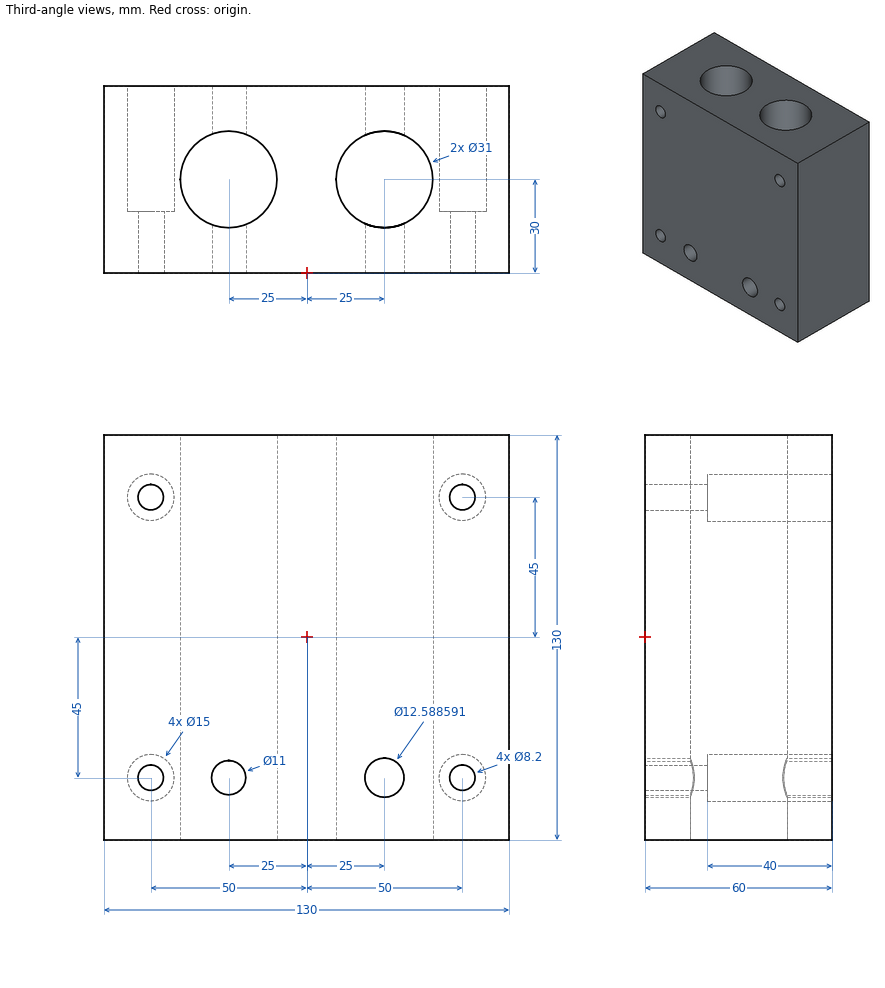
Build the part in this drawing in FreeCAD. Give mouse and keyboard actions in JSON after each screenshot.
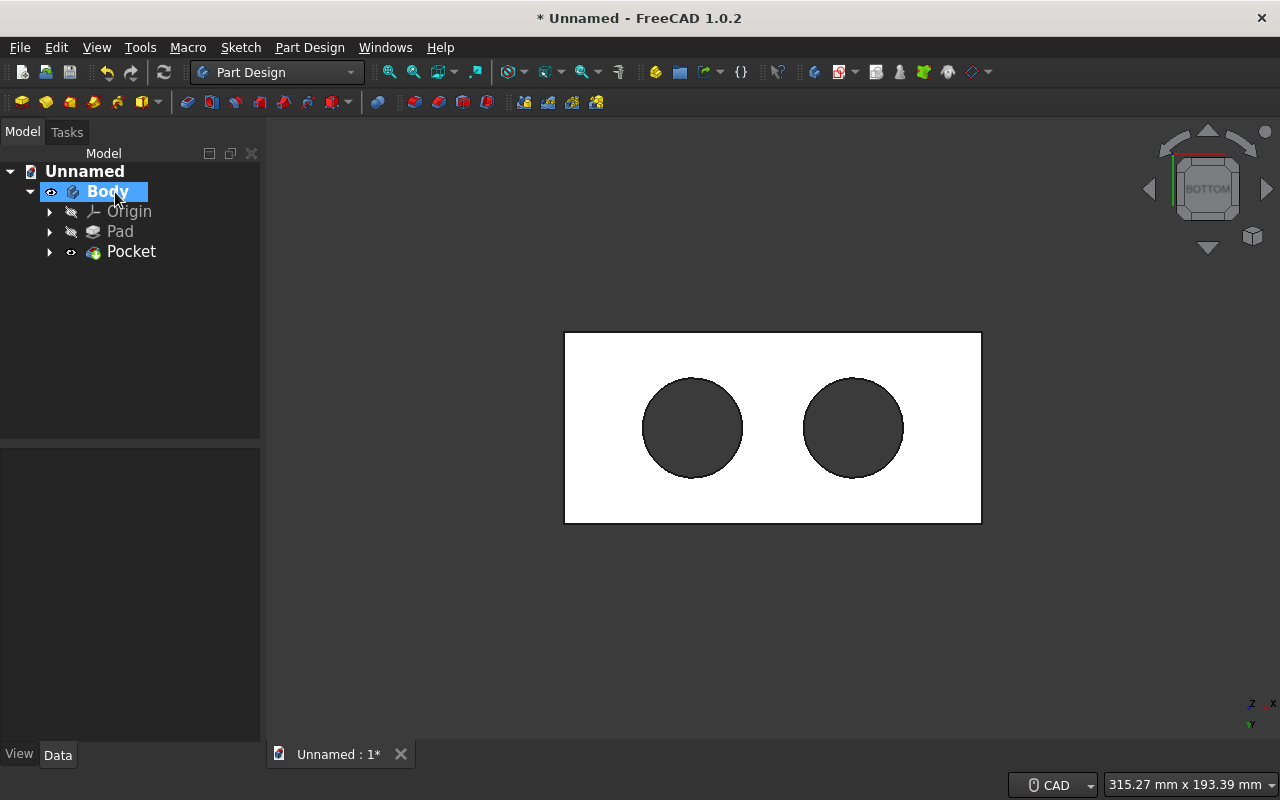
{"action": "key", "text": "4"}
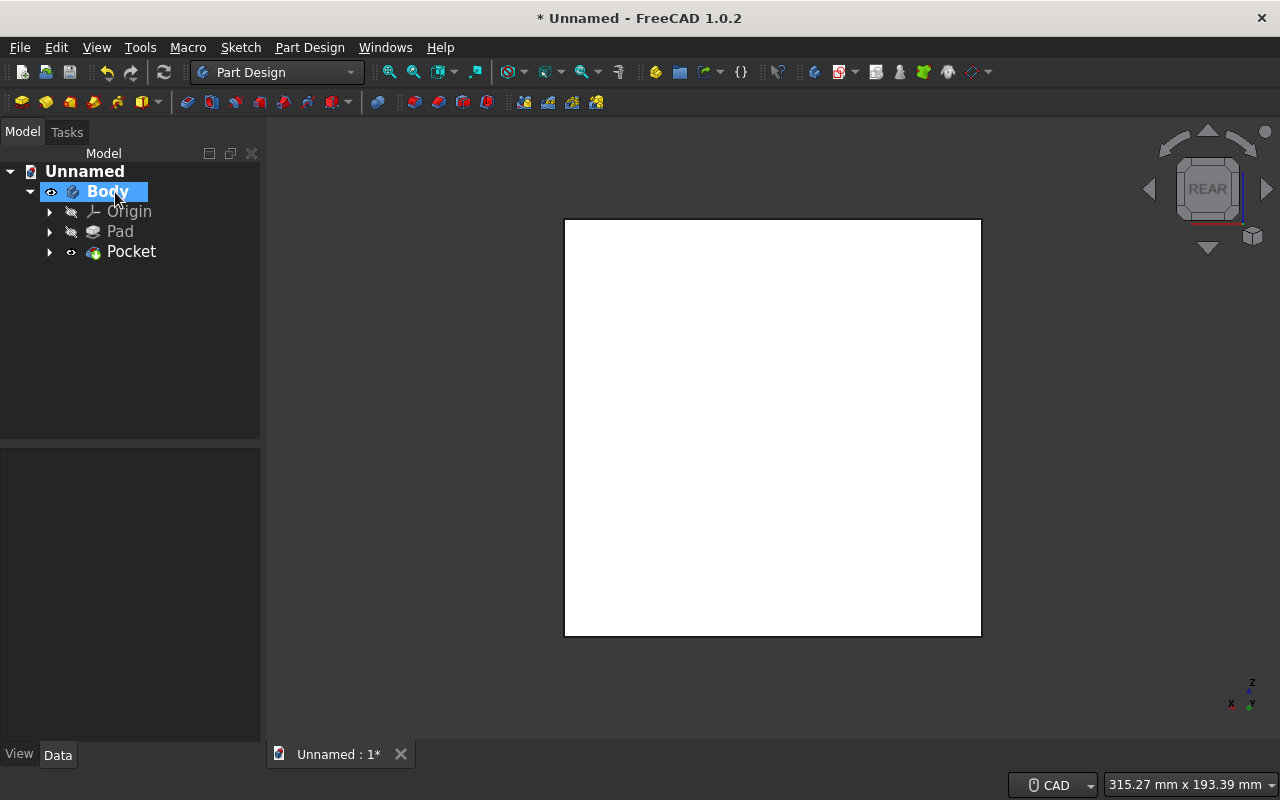
{"action": "left_click", "coordinate": [773, 427]}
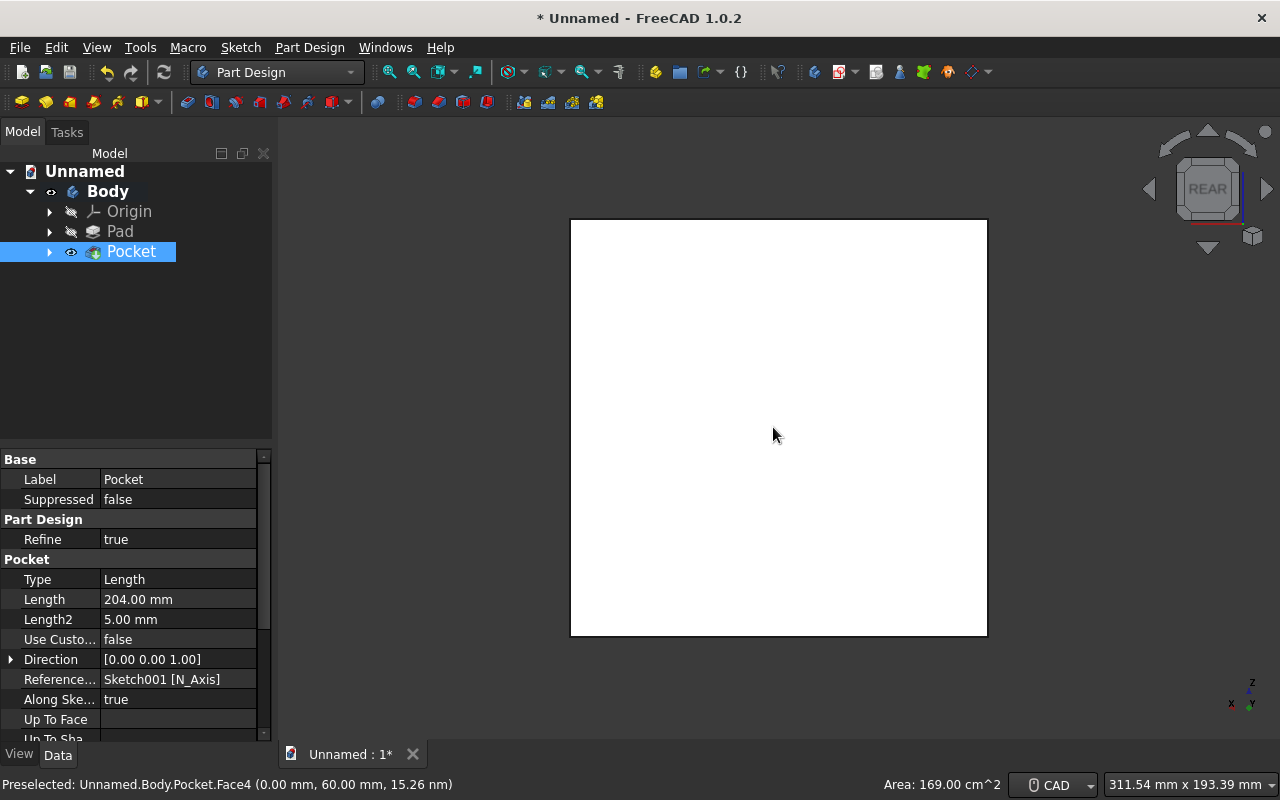
{"action": "left_click", "coordinate": [840, 72]}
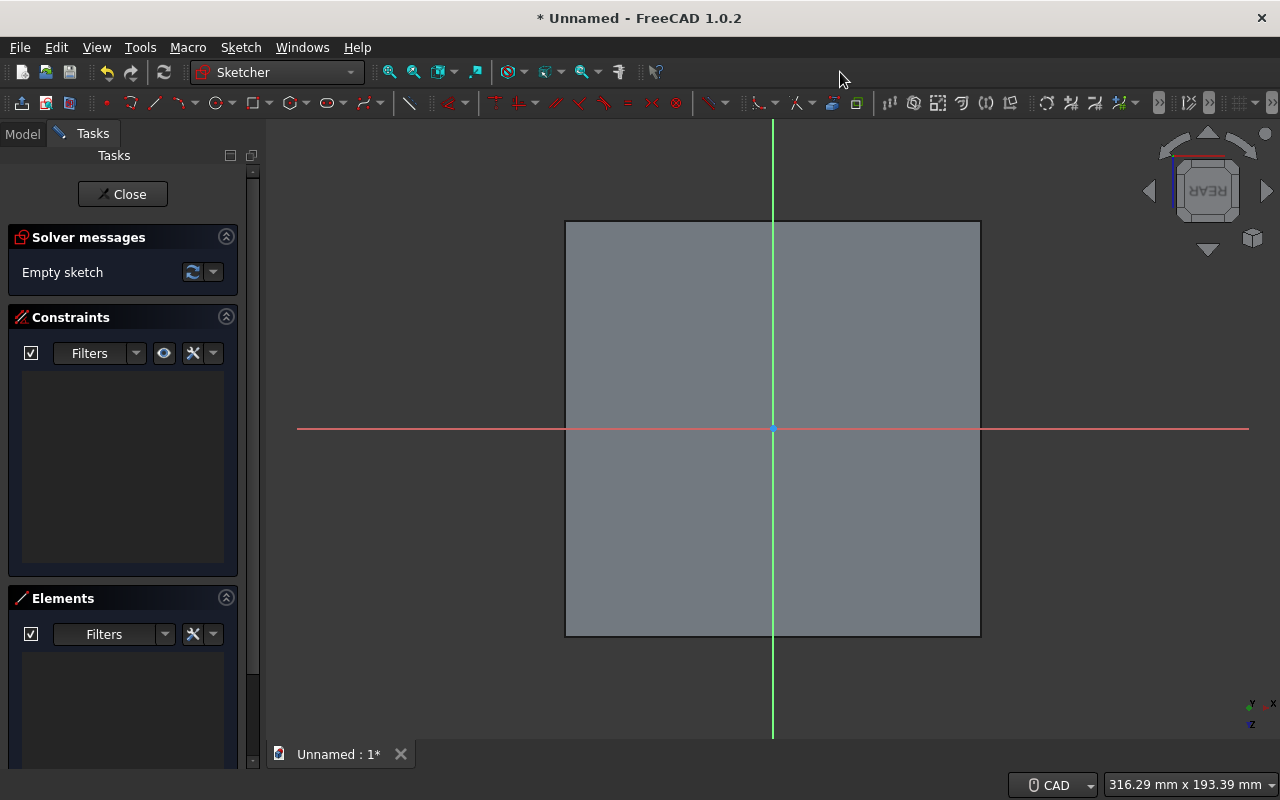
{"action": "key", "text": "g c"}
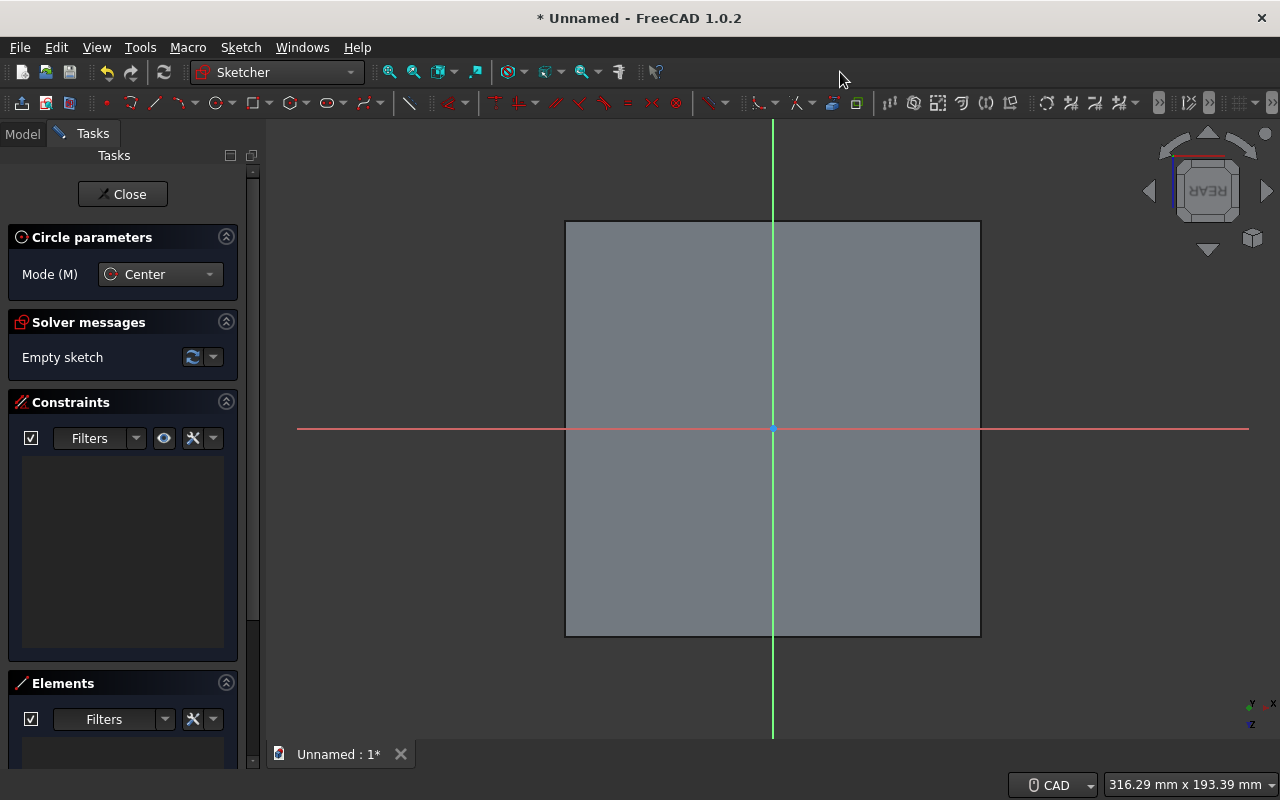
{"action": "left_click", "coordinate": [613, 285]}
{"action": "left_click", "coordinate": [630, 268]}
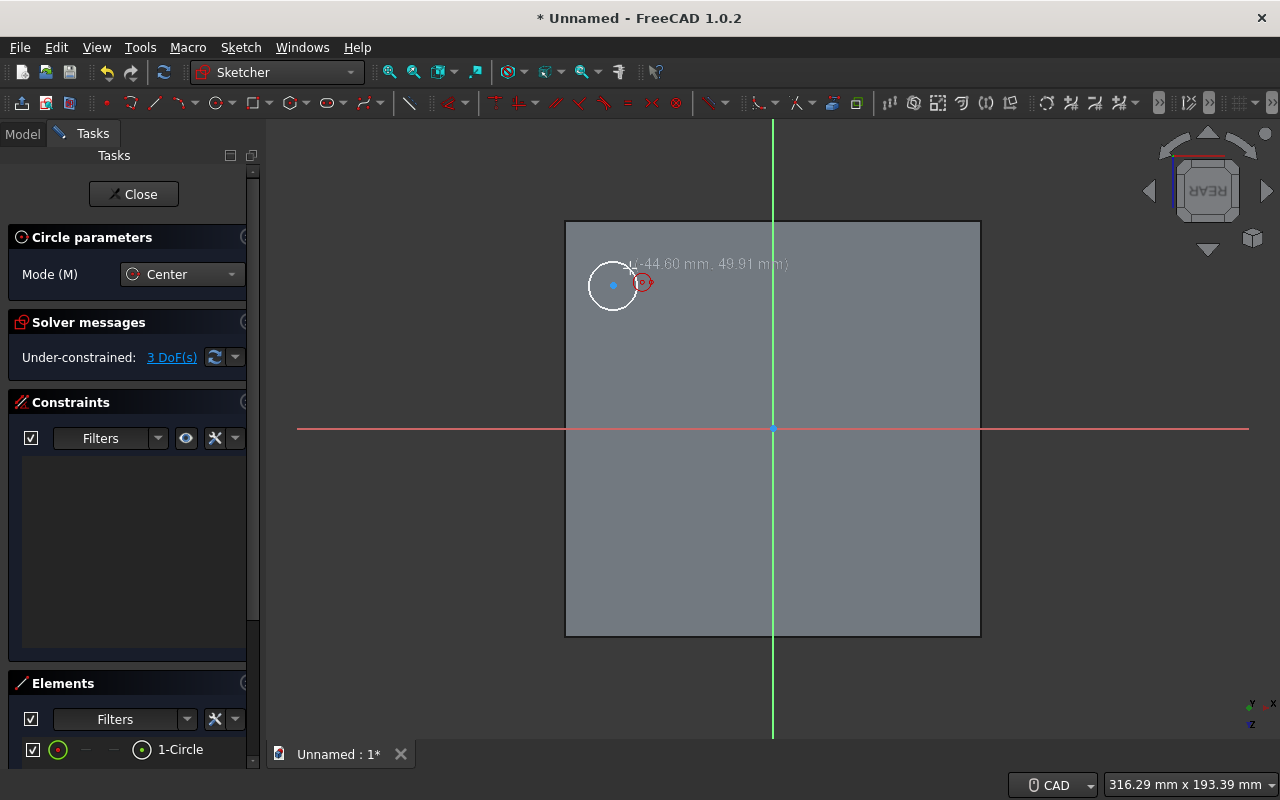
{"action": "left_click", "coordinate": [933, 285]}
{"action": "left_click", "coordinate": [950, 268]}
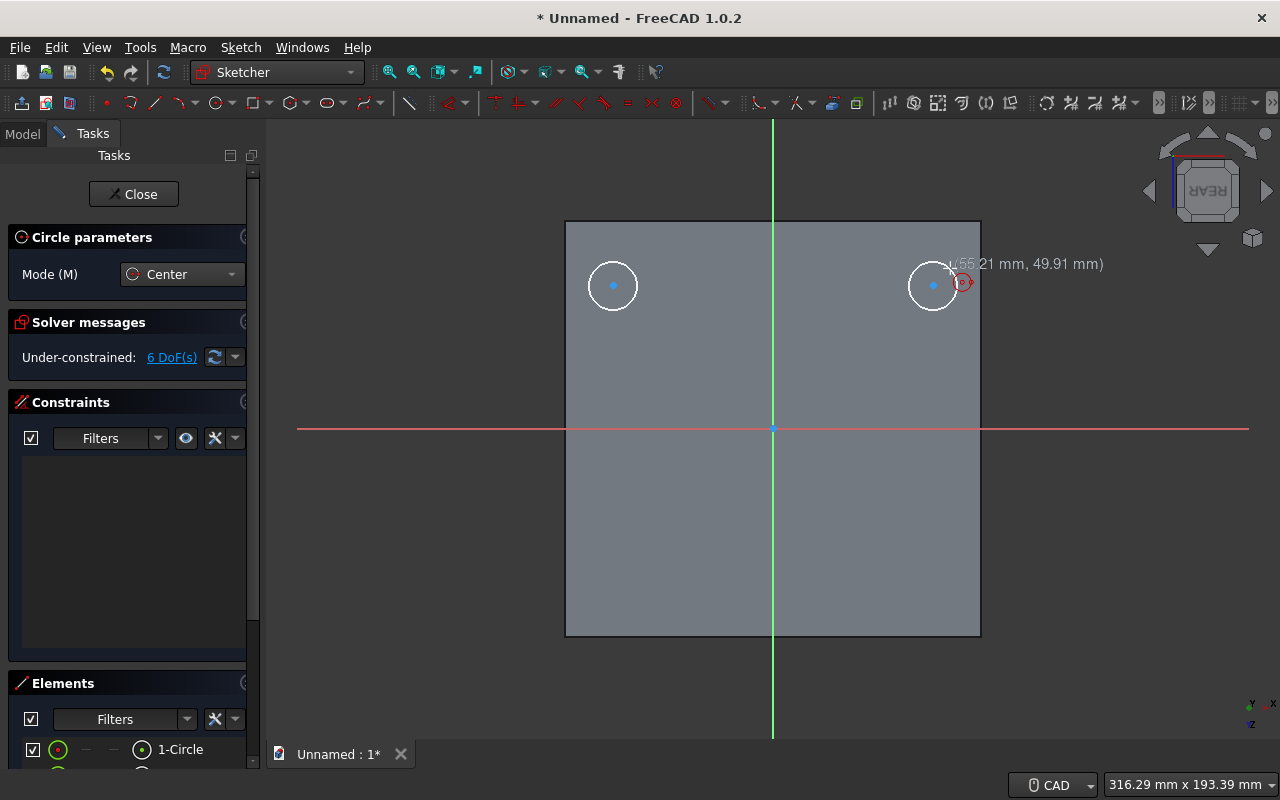
{"action": "left_click", "coordinate": [933, 573]}
{"action": "left_click", "coordinate": [950, 556]}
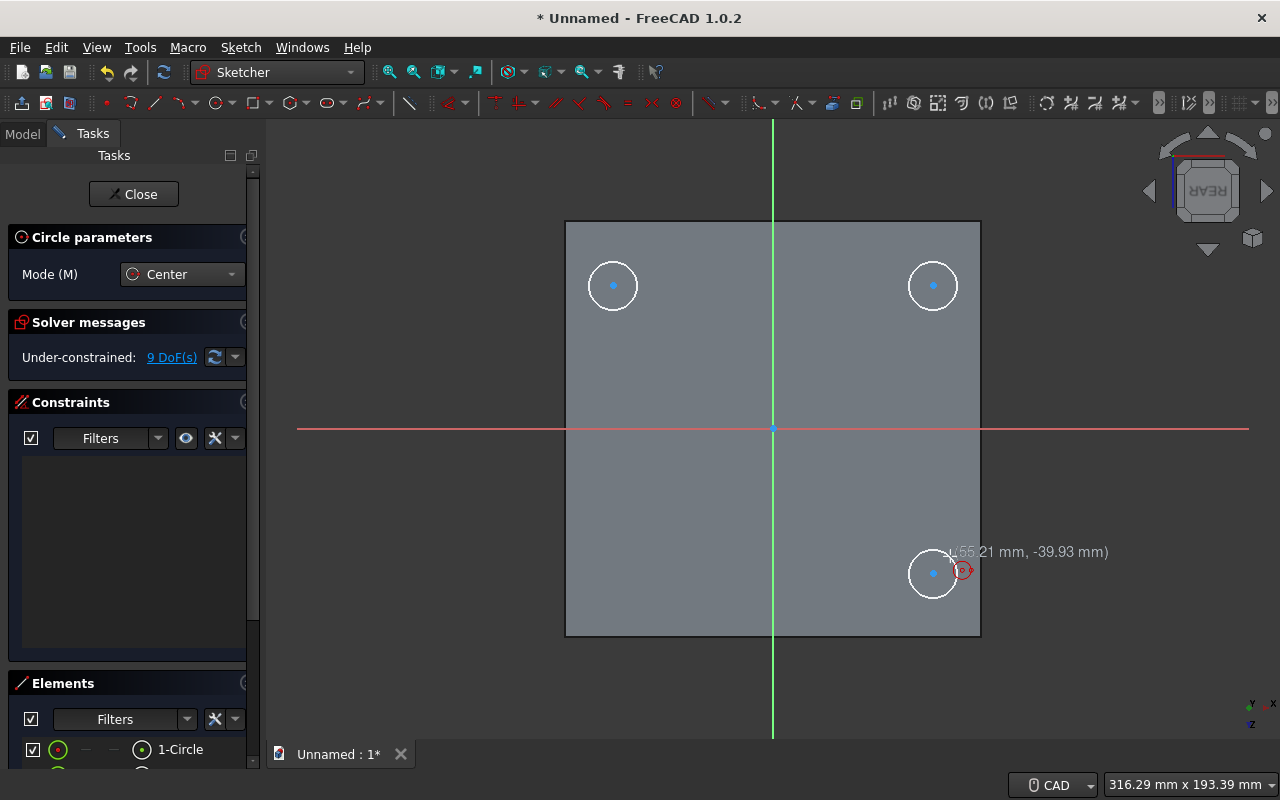
{"action": "left_click", "coordinate": [613, 573]}
{"action": "left_click", "coordinate": [630, 556]}
{"action": "key", "text": "Escape"}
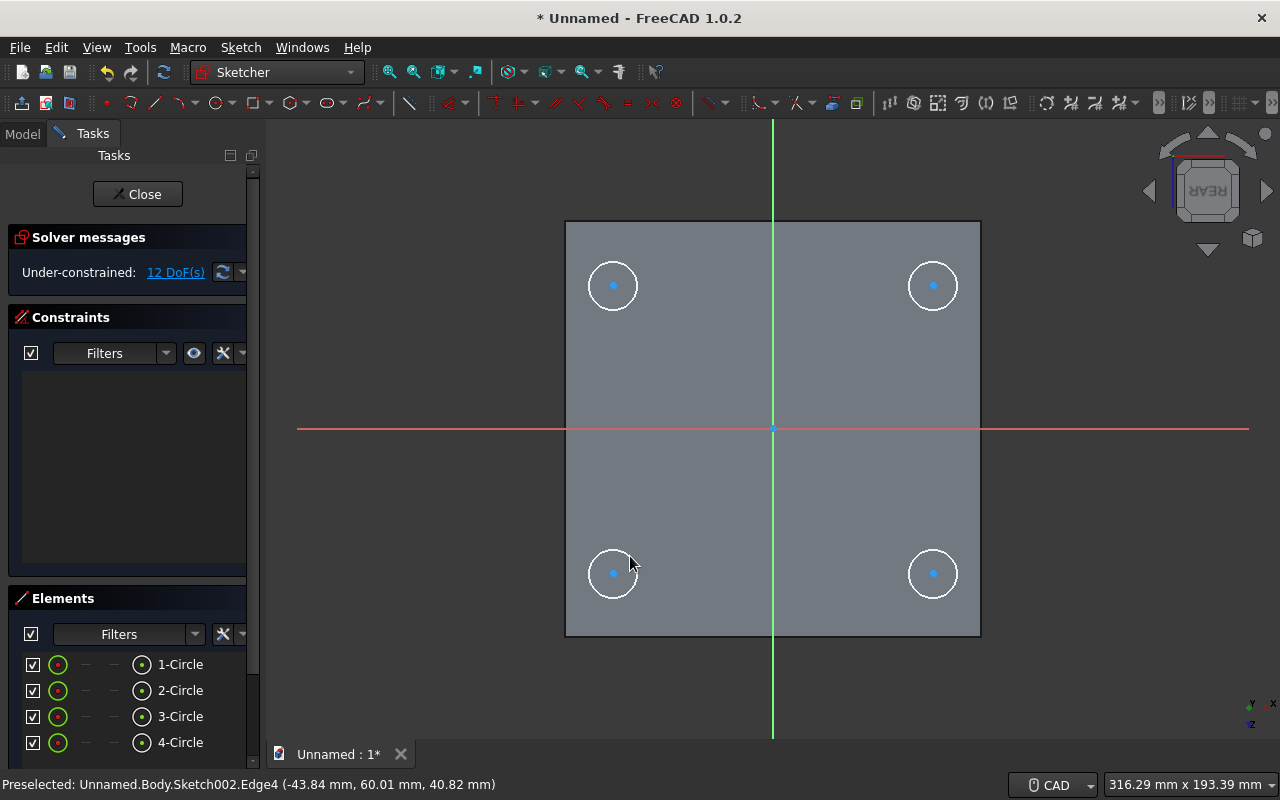
{"action": "left_click", "coordinate": [630, 269]}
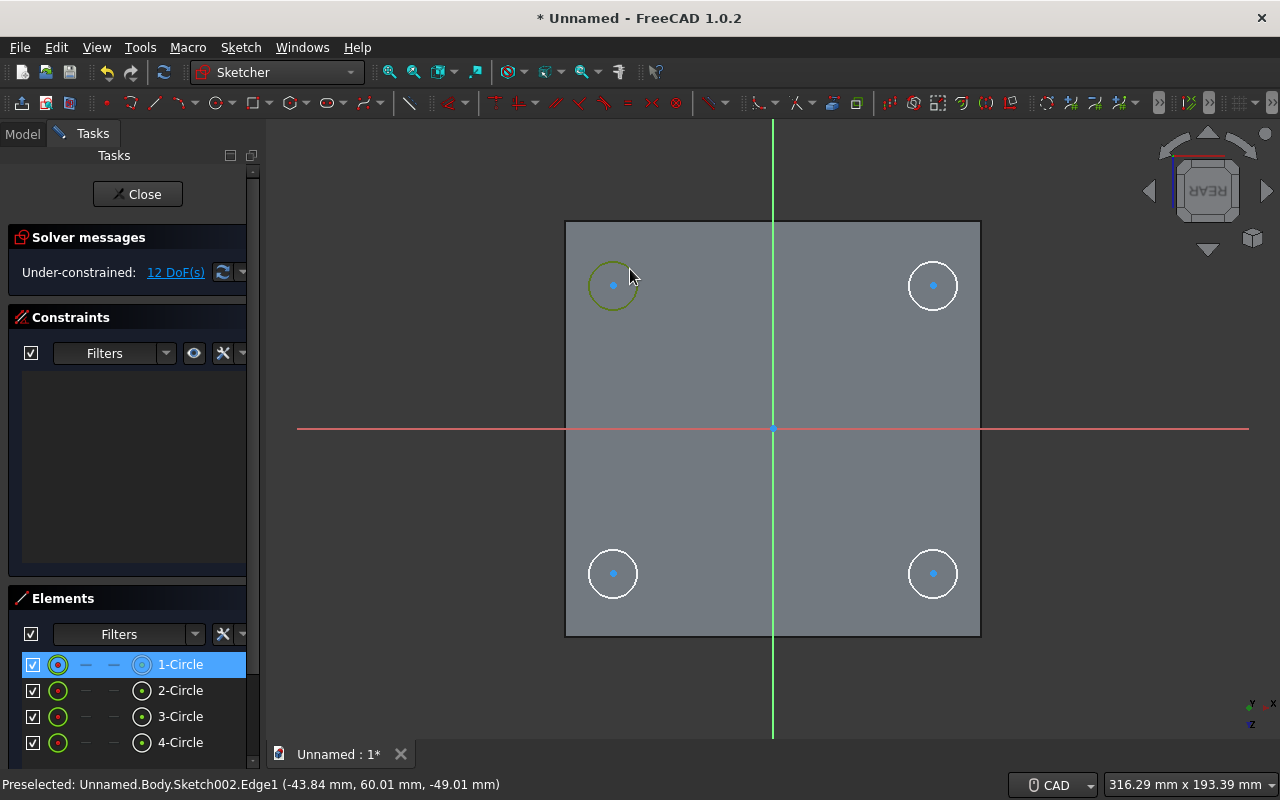
{"action": "left_click", "coordinate": [950, 269]}